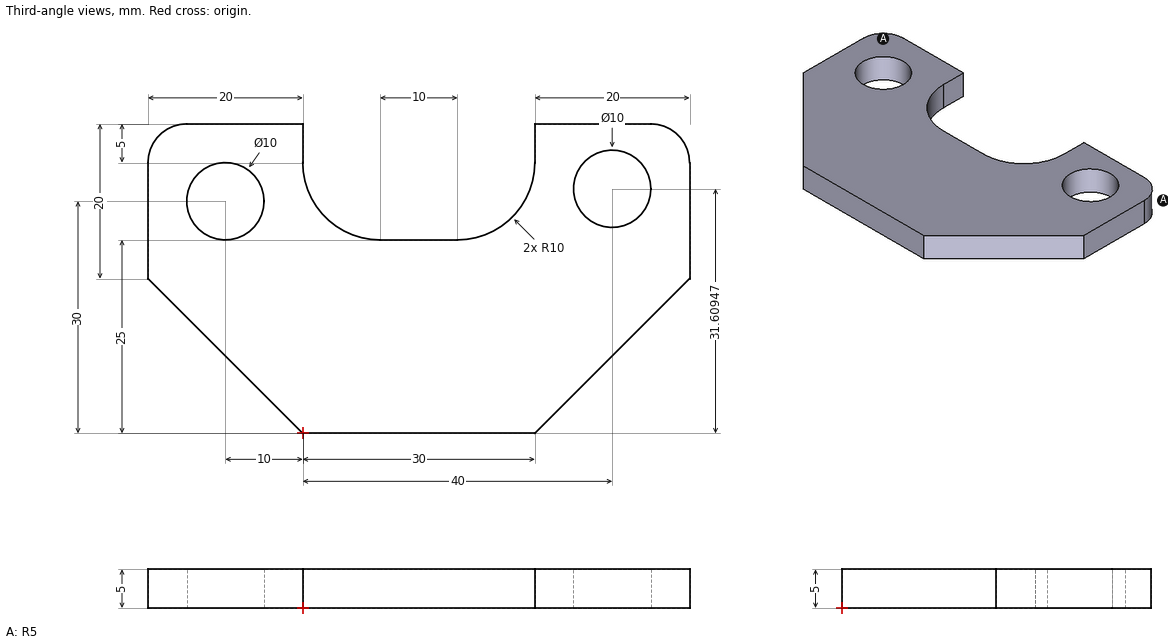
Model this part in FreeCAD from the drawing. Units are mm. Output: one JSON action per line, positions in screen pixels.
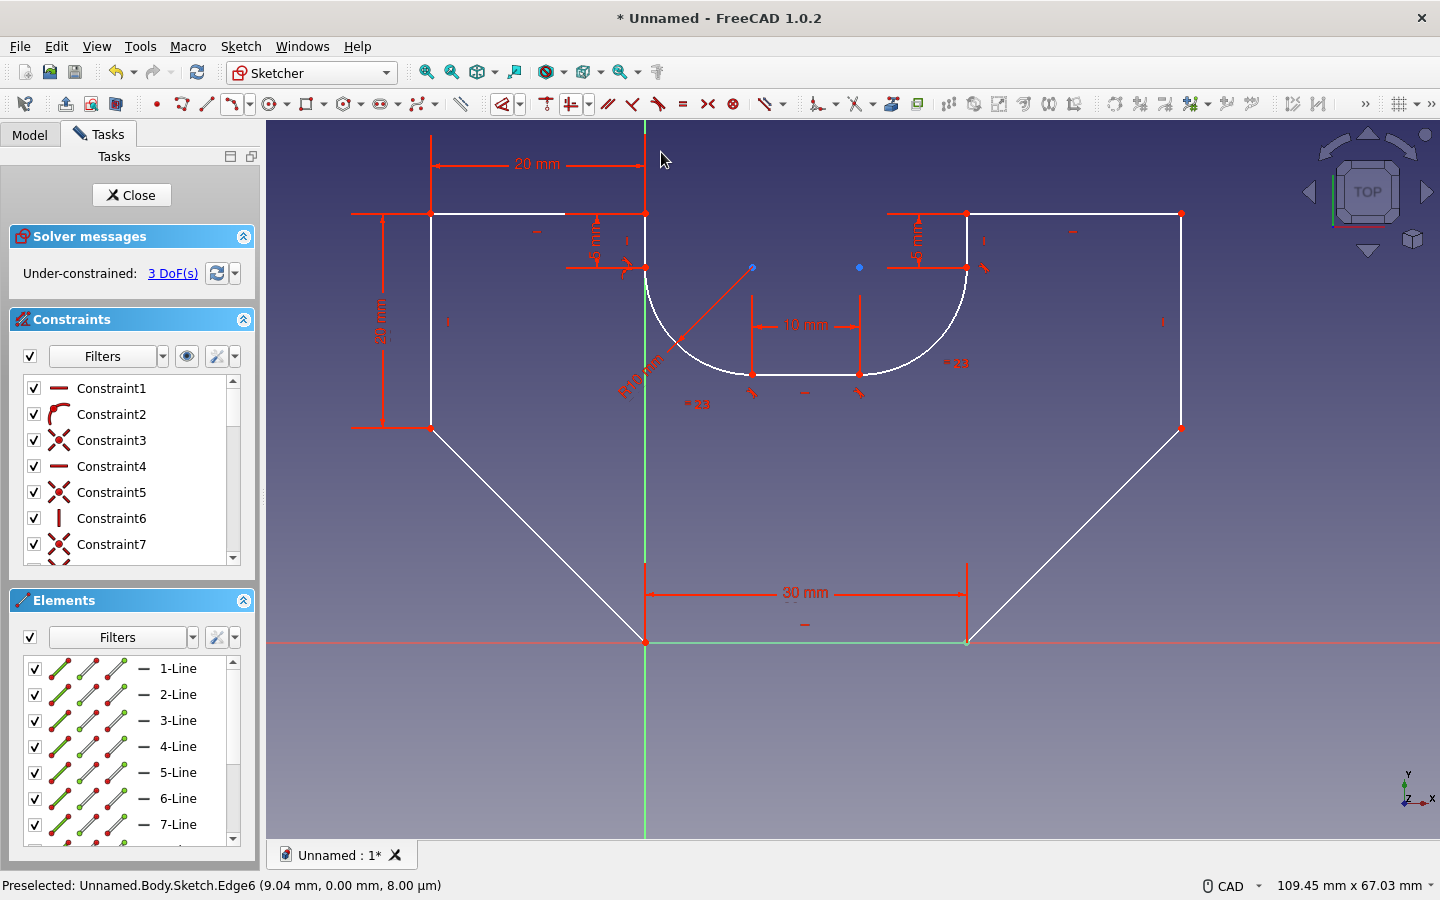
{"action": "left_click", "coordinate": [1181, 364]}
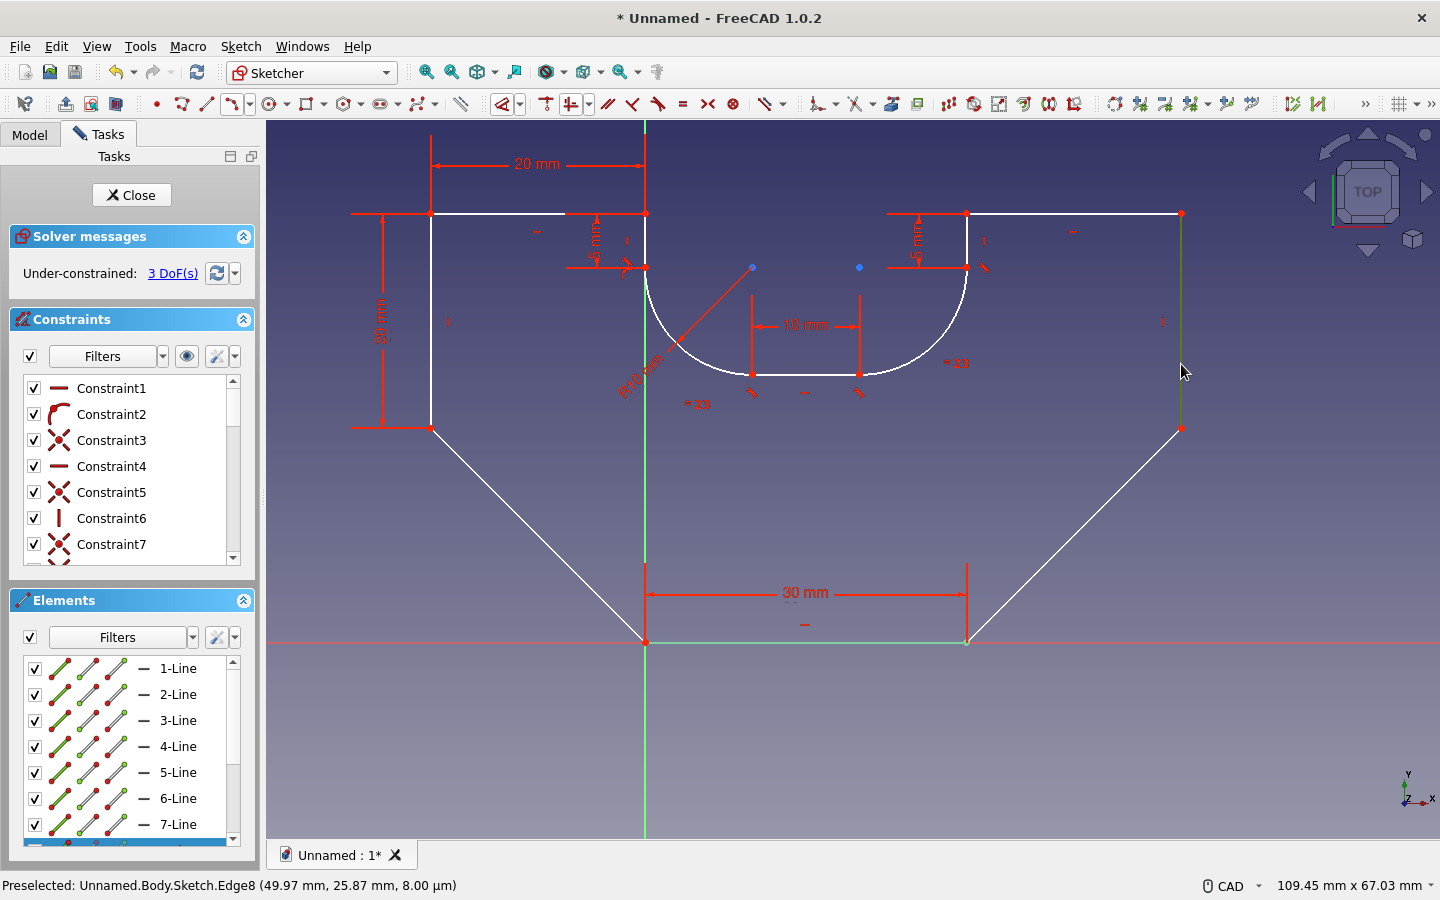
{"action": "left_click", "coordinate": [520, 104]}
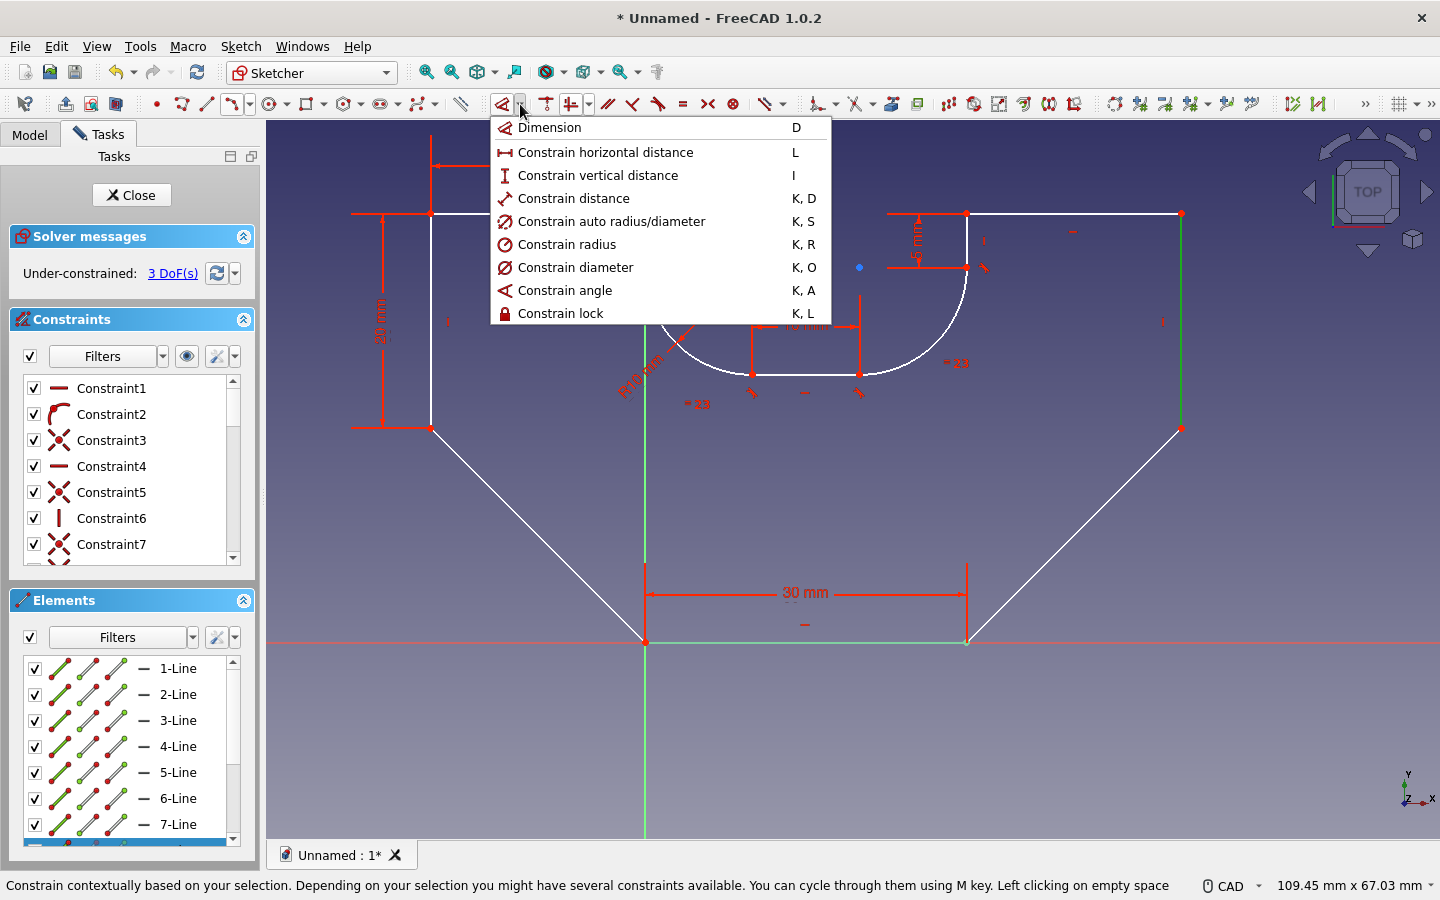
{"action": "left_click", "coordinate": [661, 176]}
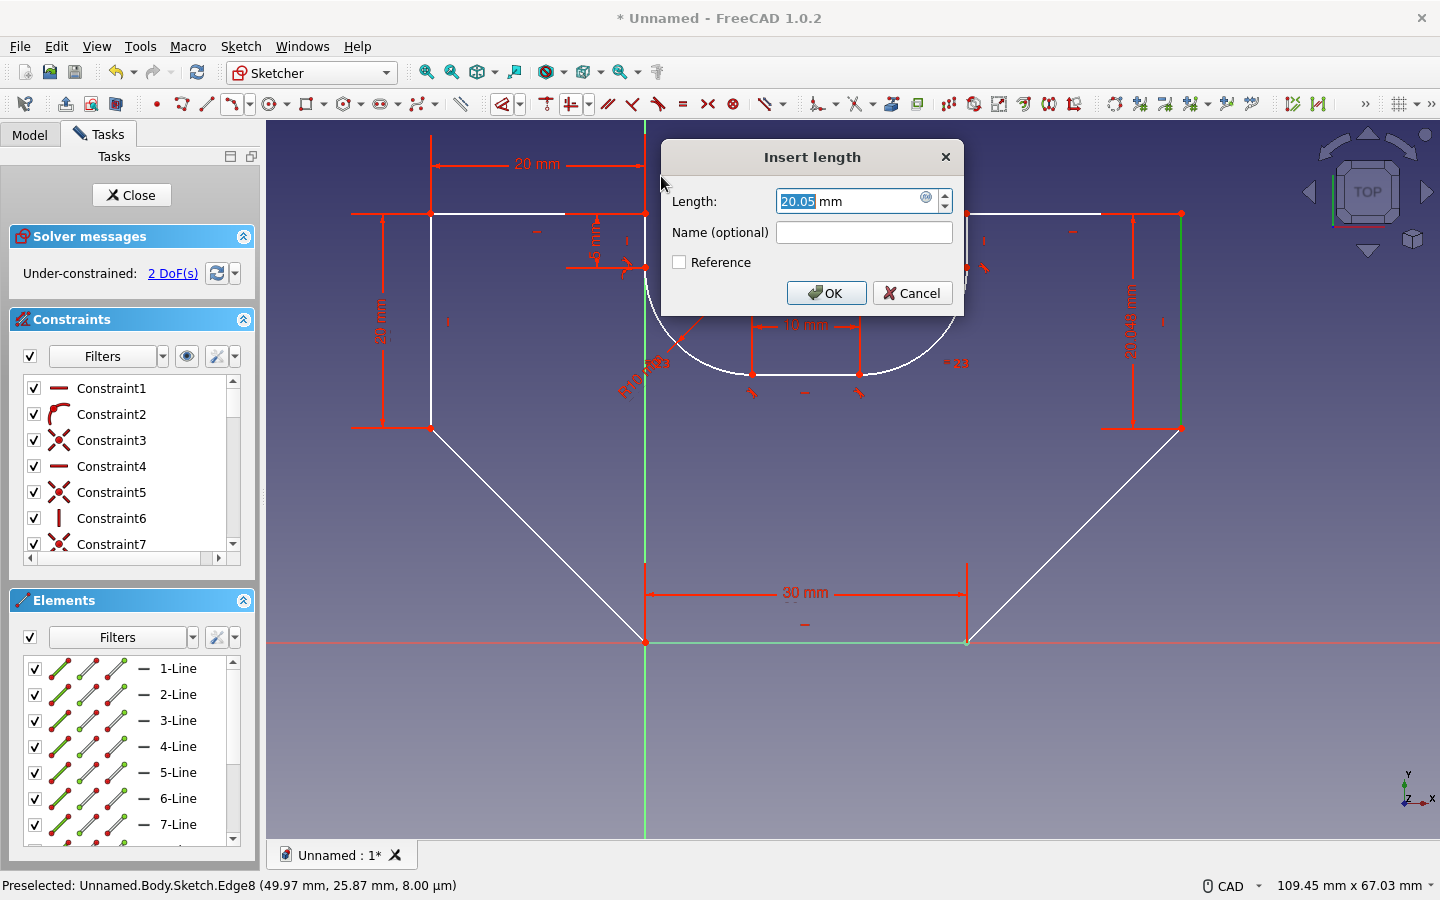
{"action": "type", "text": "20"}
{"action": "key", "text": "Return"}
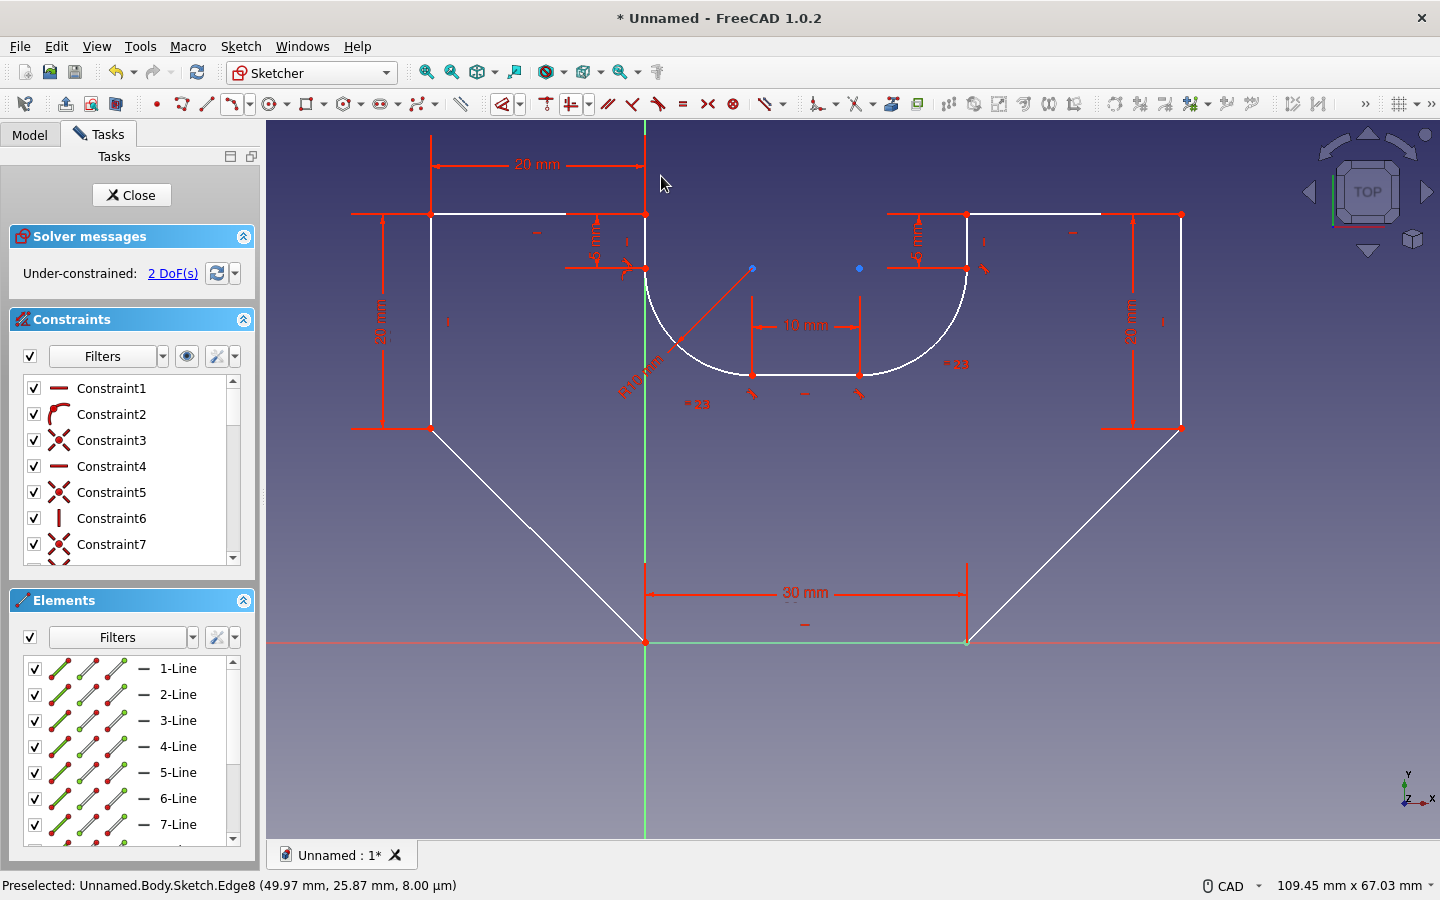
{"action": "left_click", "coordinate": [1117, 214]}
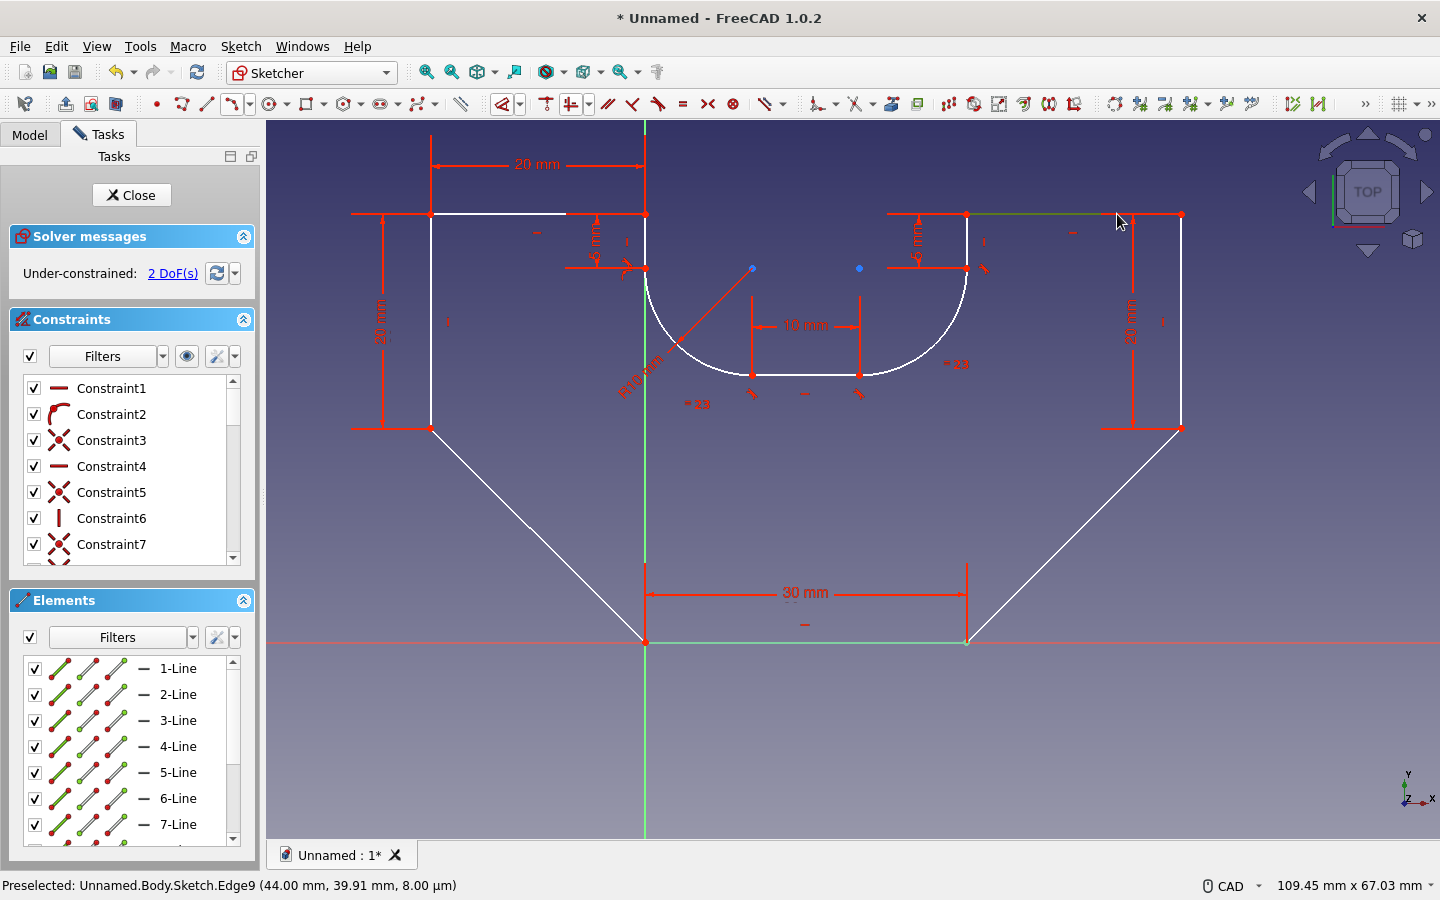
{"action": "left_click", "coordinate": [520, 104]}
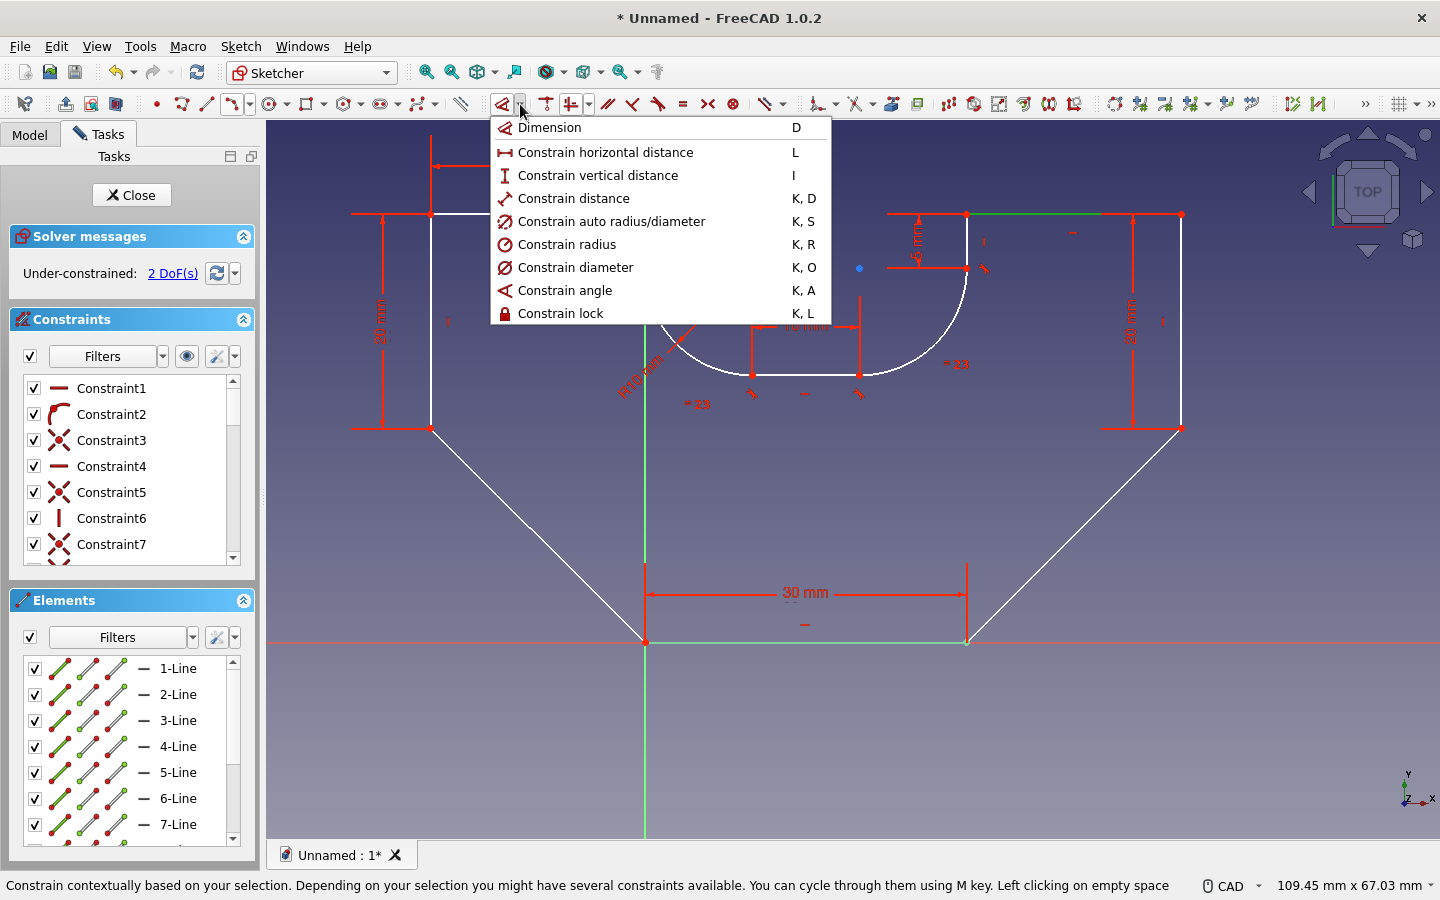
{"action": "left_click", "coordinate": [661, 152]}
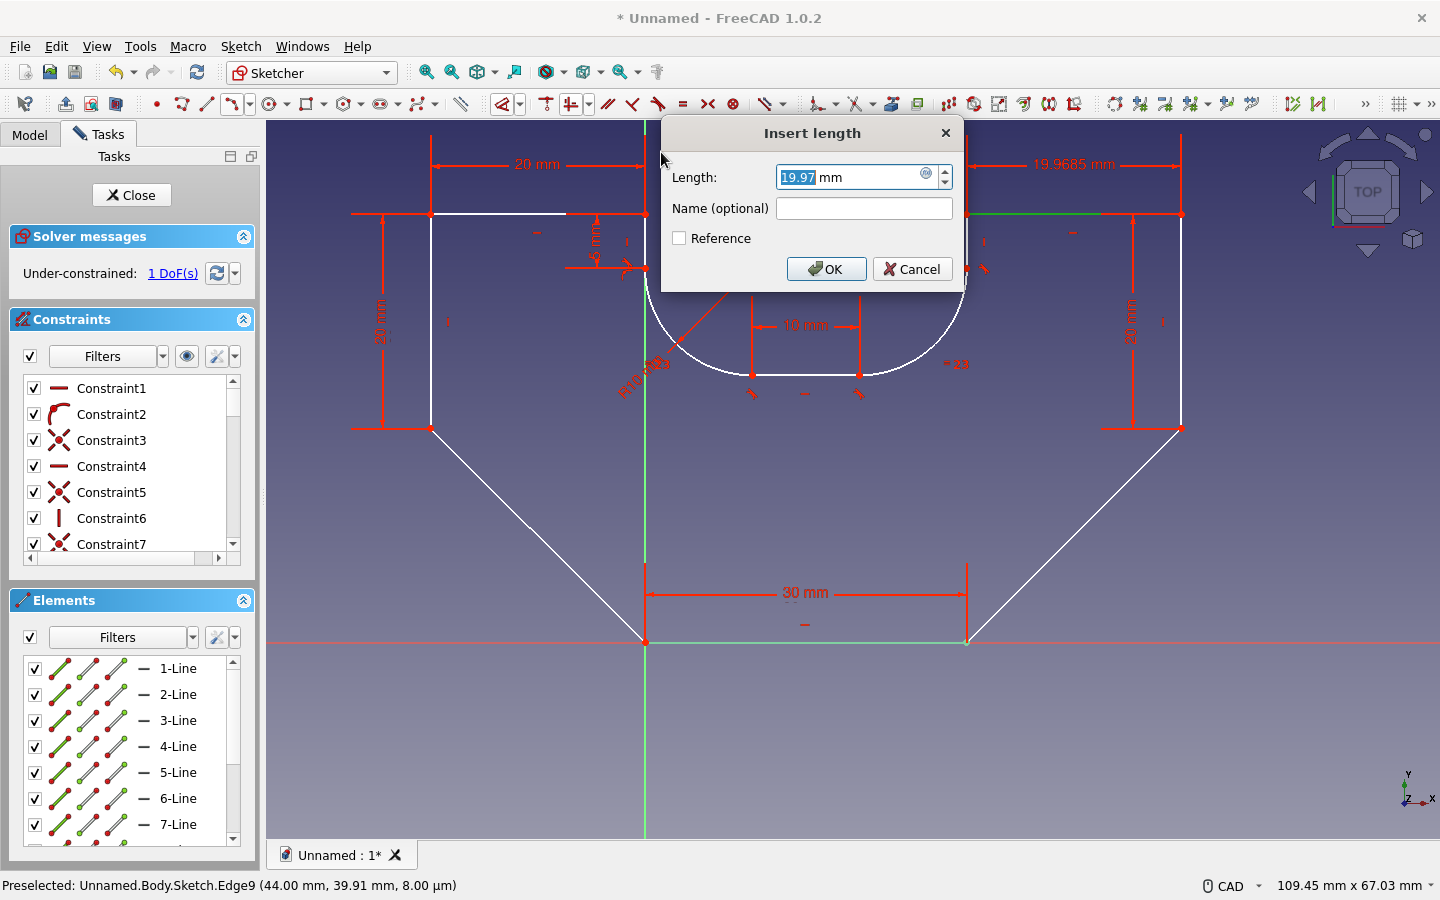
{"action": "type", "text": "20"}
{"action": "key", "text": "Return"}